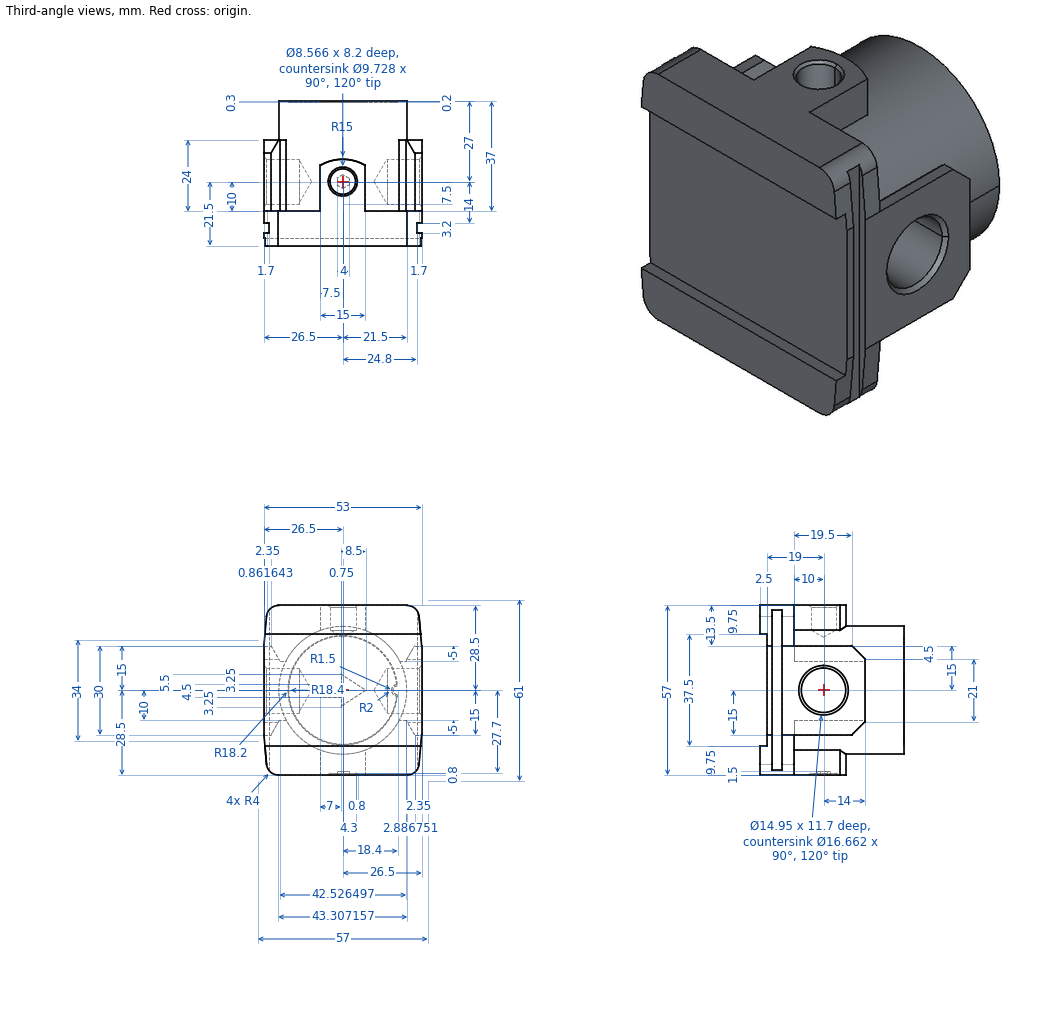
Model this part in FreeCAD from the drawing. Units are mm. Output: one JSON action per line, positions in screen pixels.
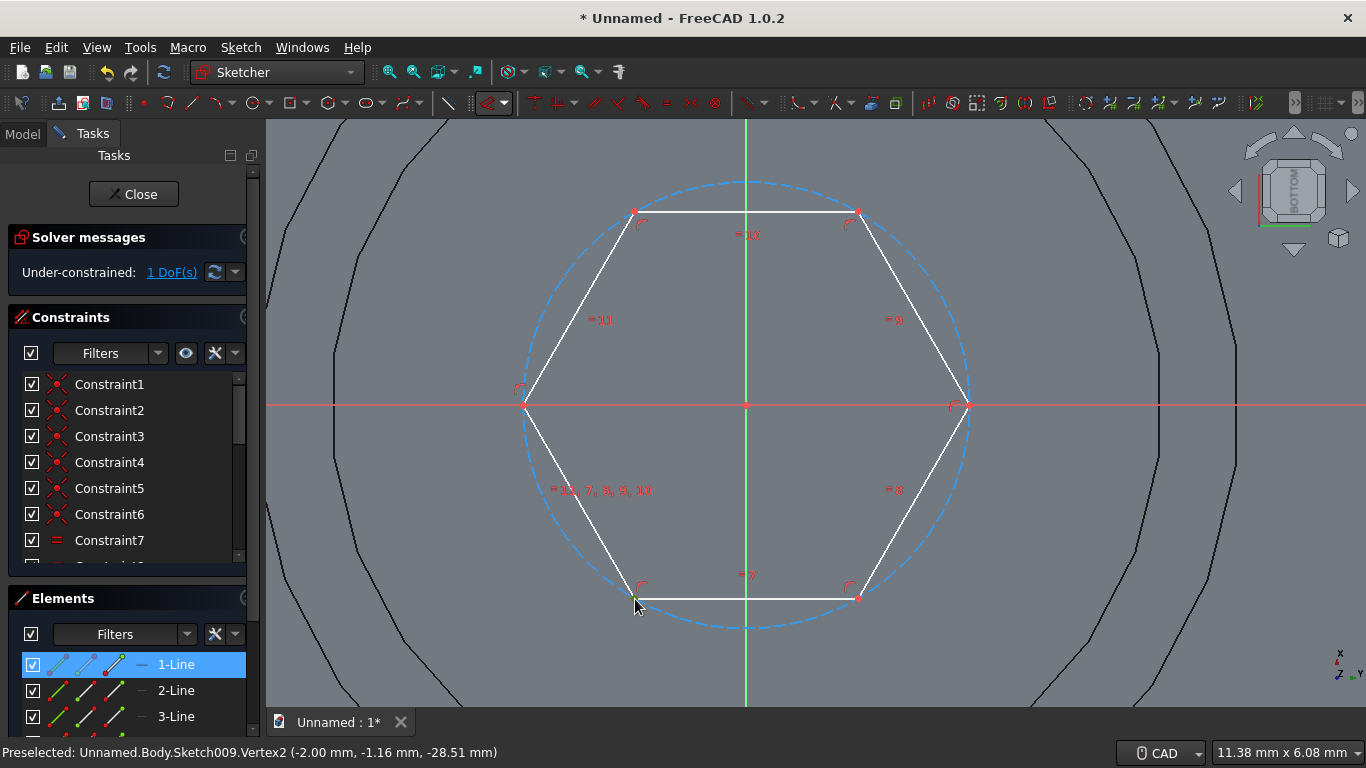
{"action": "left_click", "coordinate": [858, 212]}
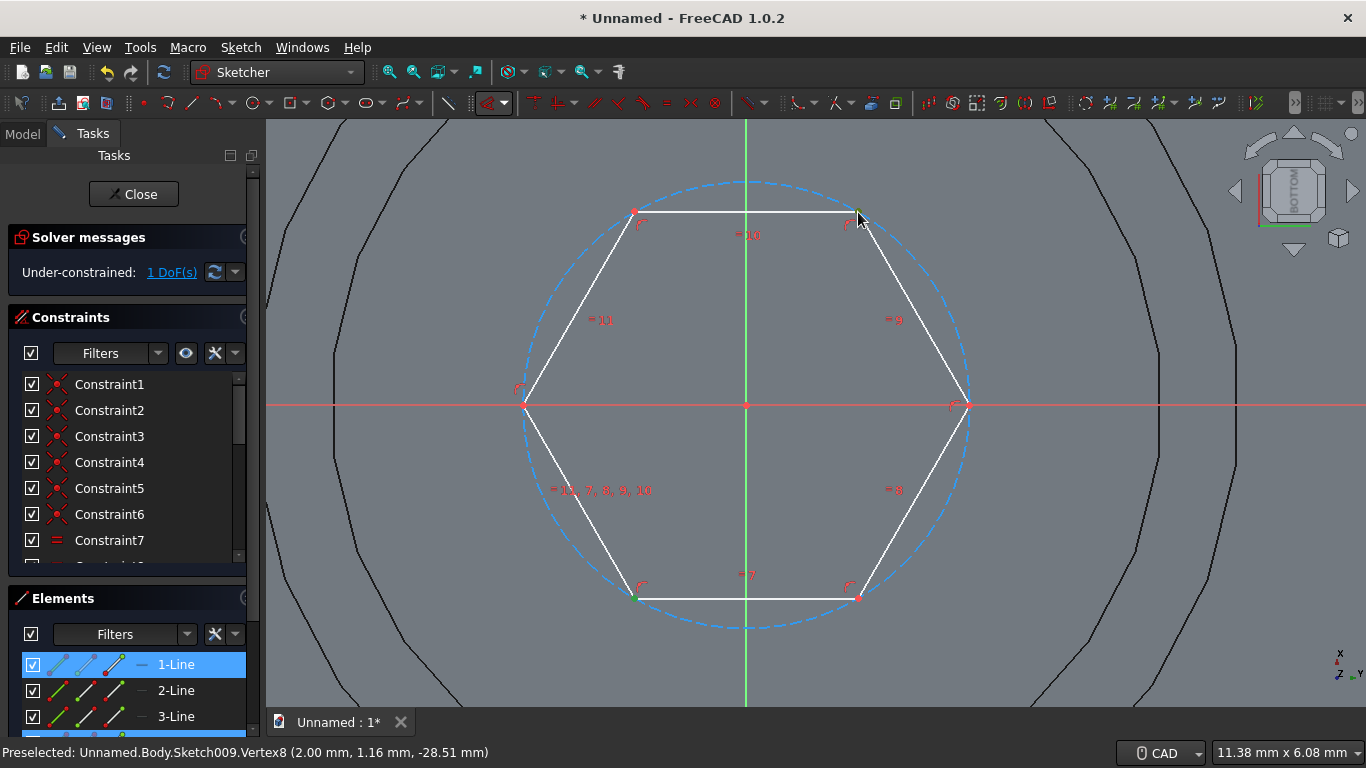
{"action": "left_click", "coordinate": [506, 104]}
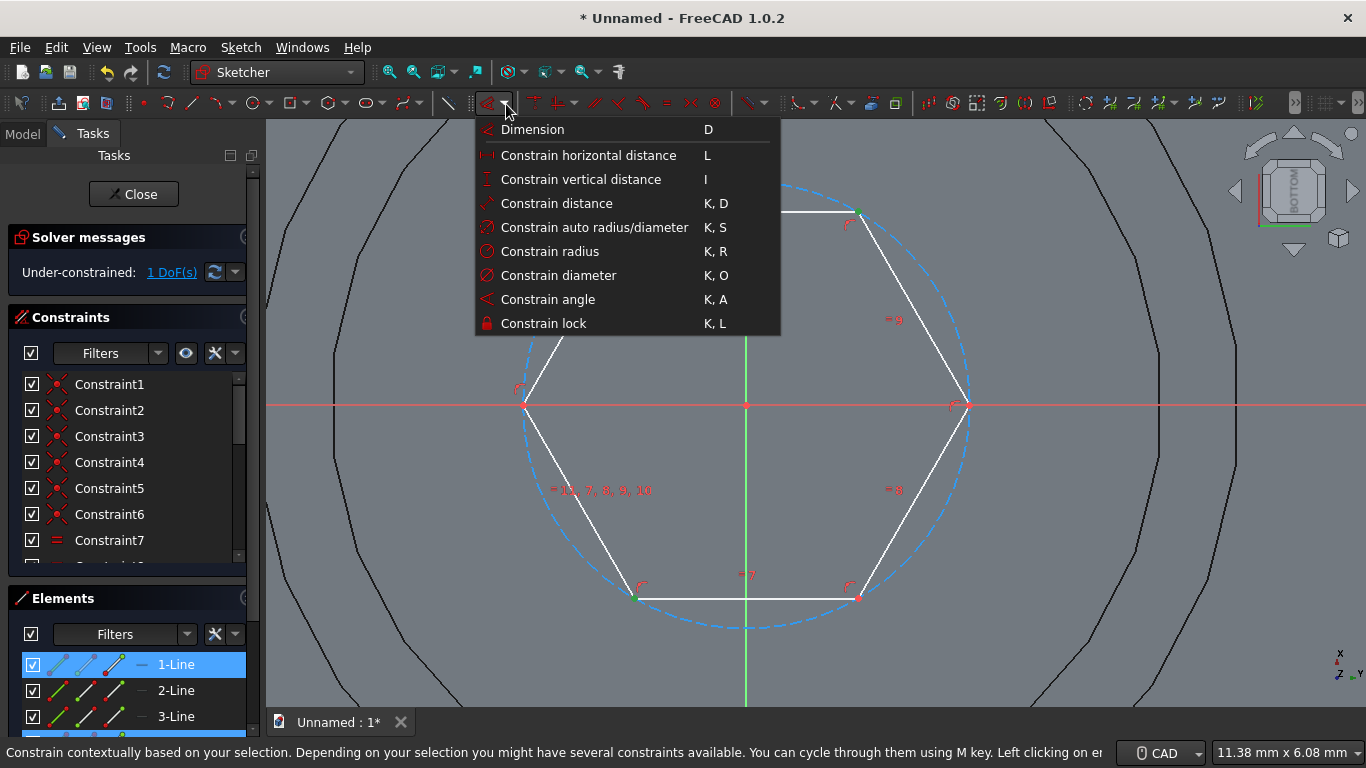
{"action": "left_click", "coordinate": [628, 179]}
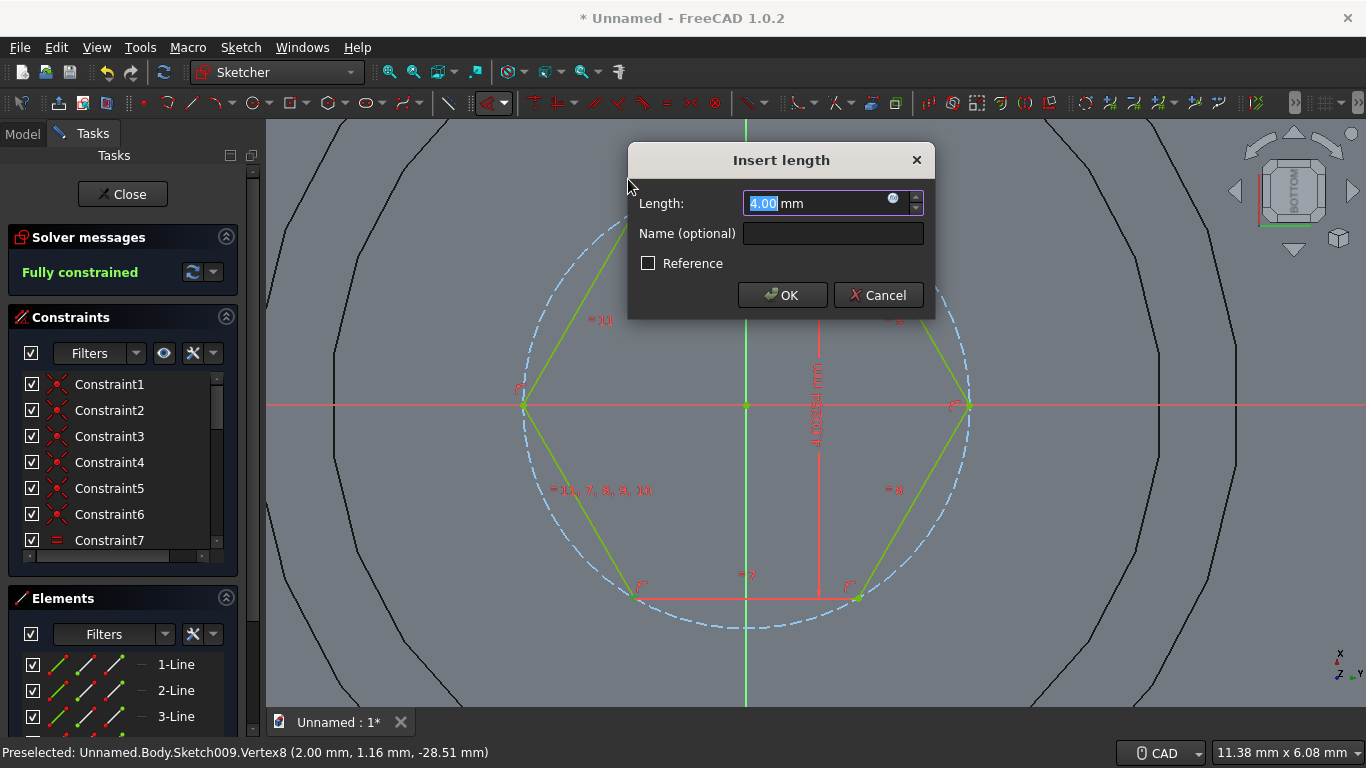
{"action": "type", "text": "4"}
{"action": "key", "text": "Return"}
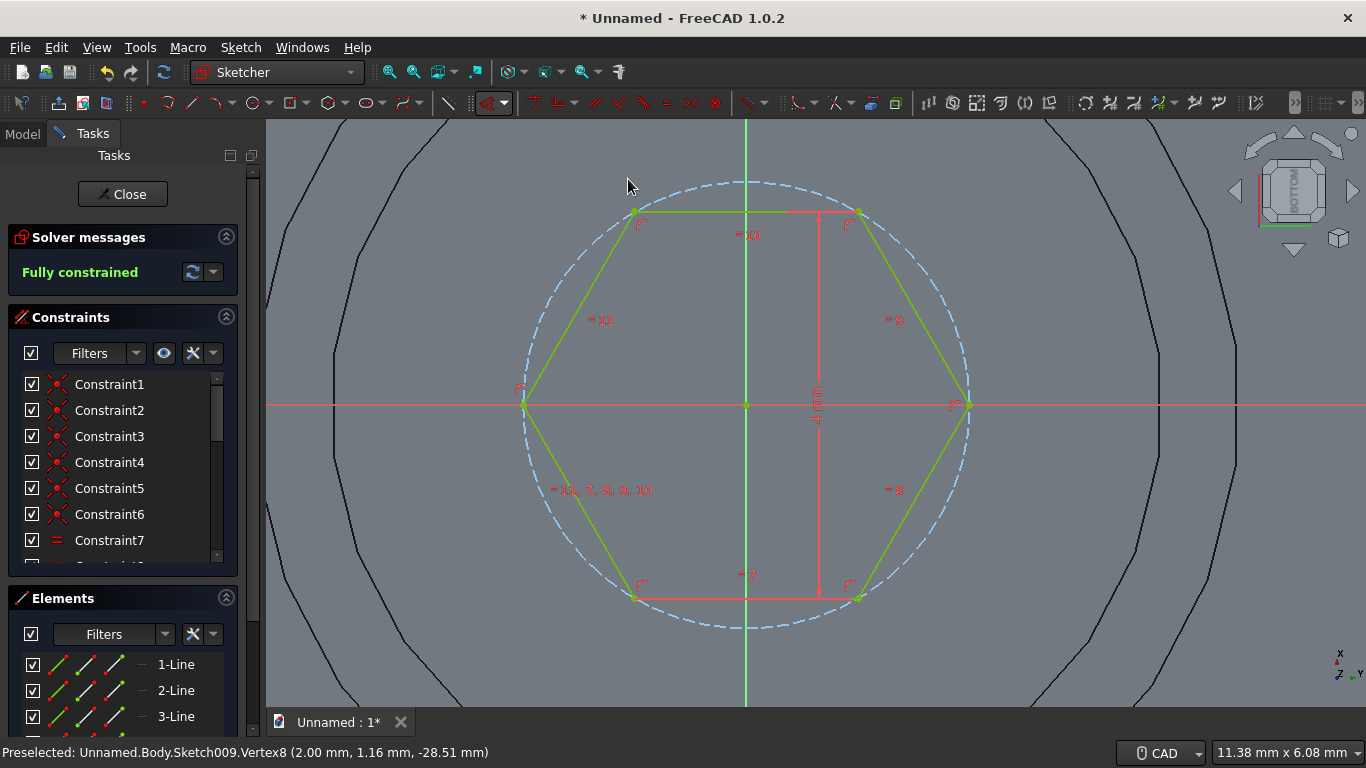
{"action": "left_click", "coordinate": [123, 194]}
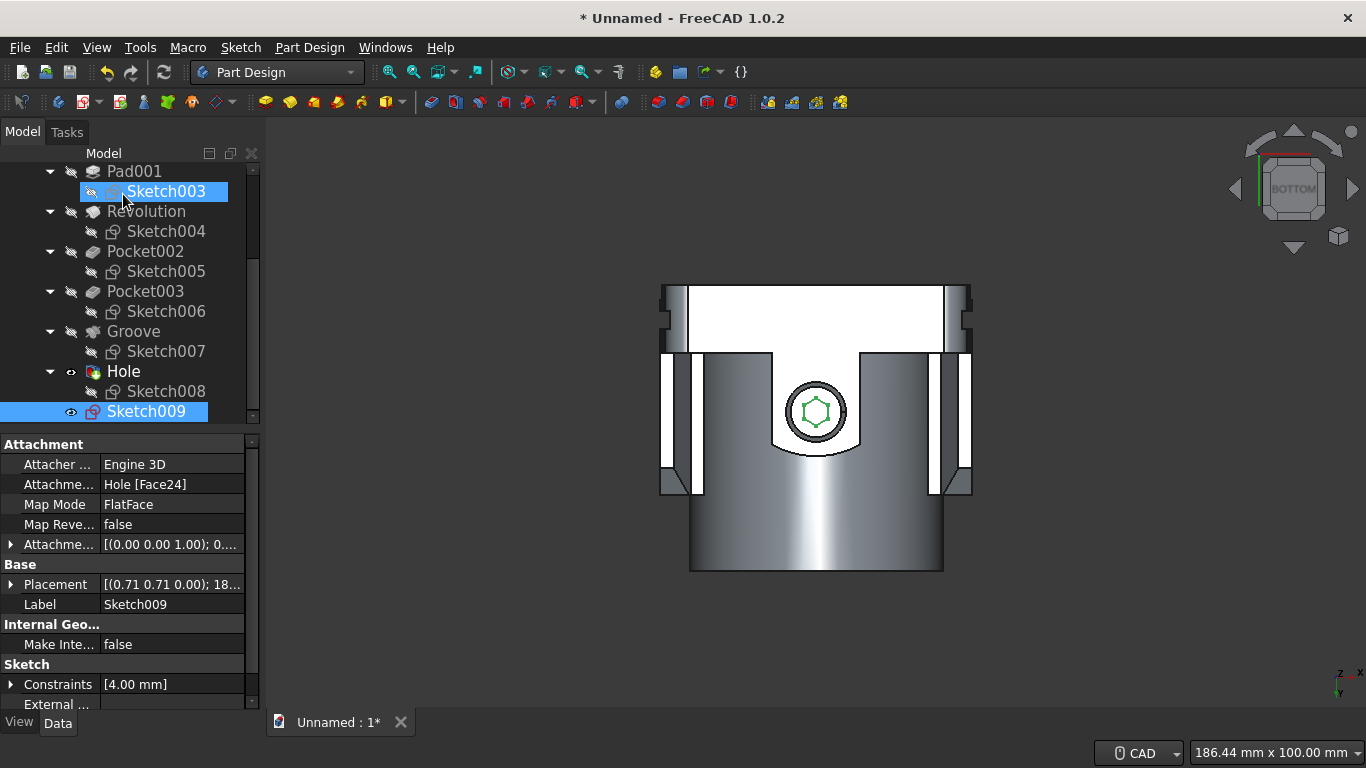
{"action": "left_click", "coordinate": [432, 102]}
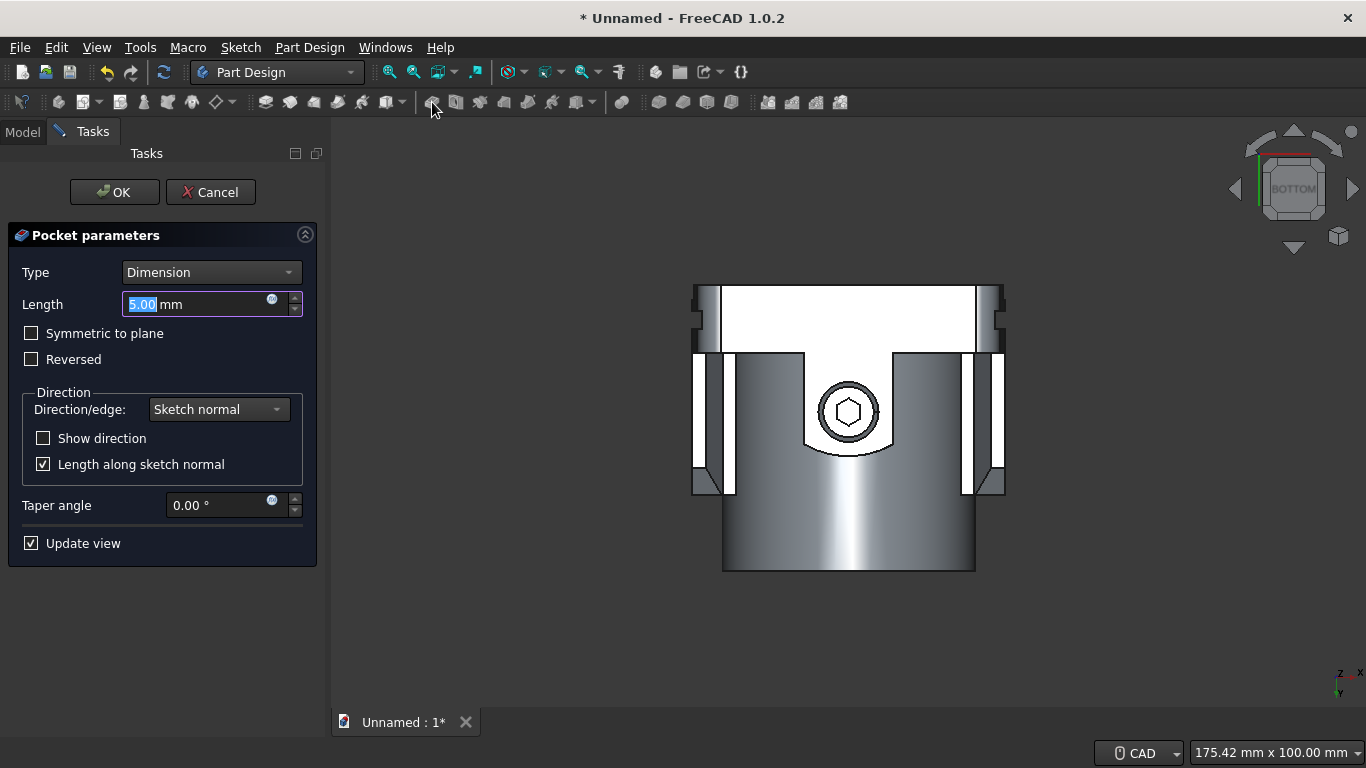
{"action": "type", "text": "1.5"}
{"action": "key", "text": "Tab"}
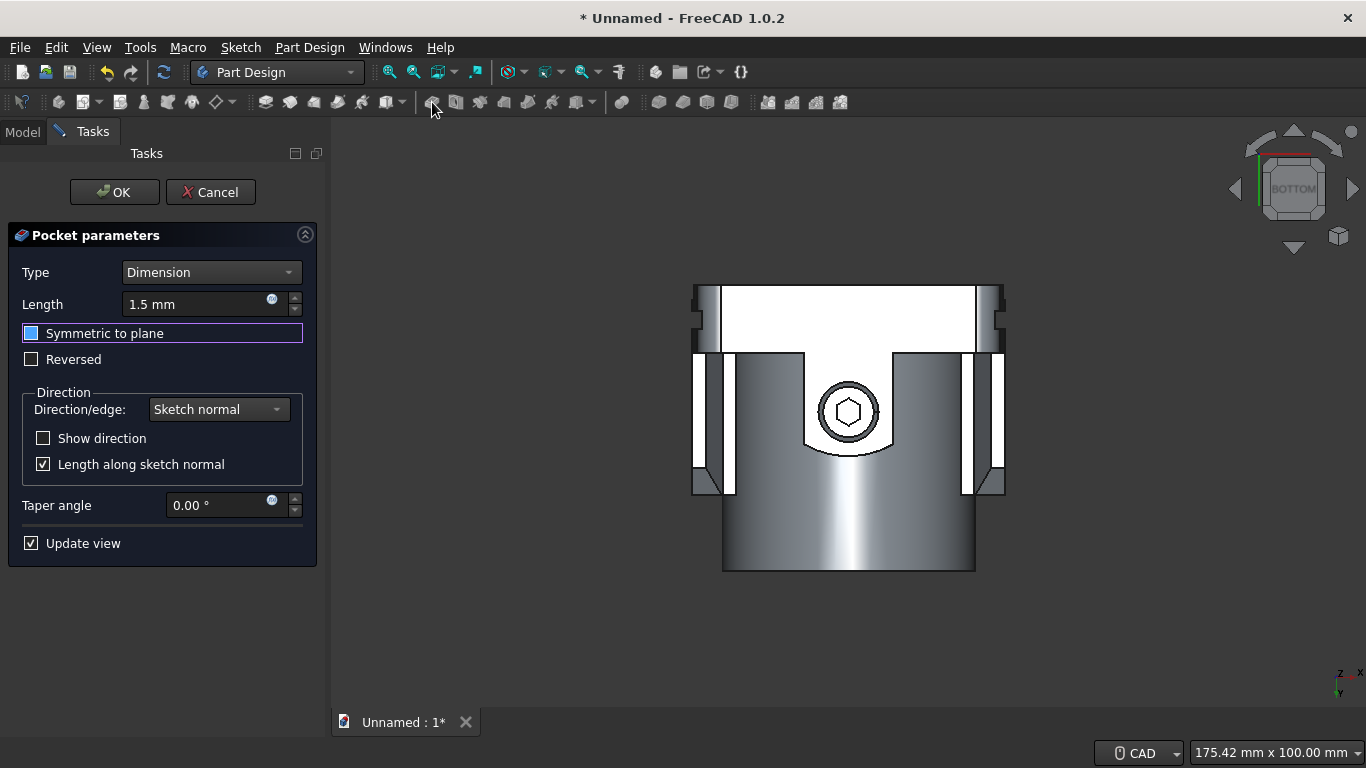
{"action": "left_click", "coordinate": [115, 192]}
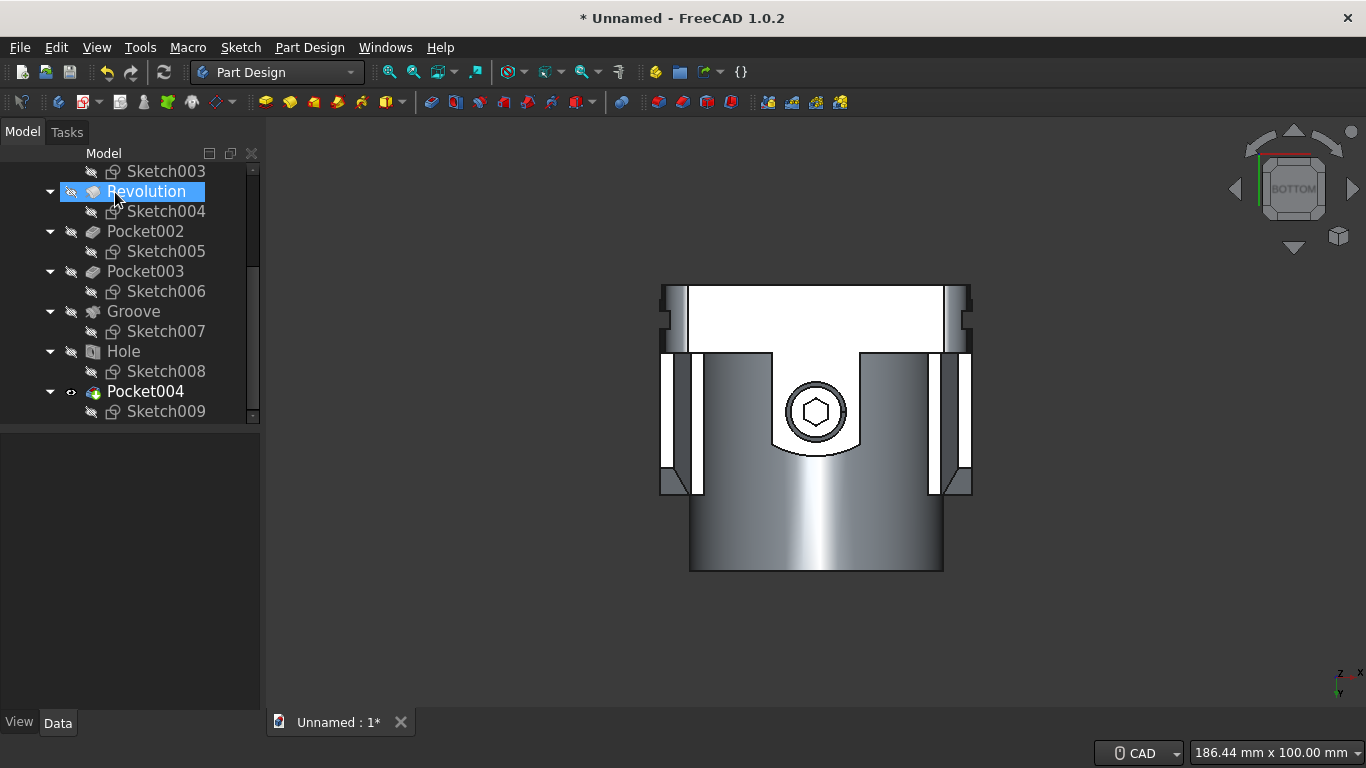
{"action": "key", "text": "0"}